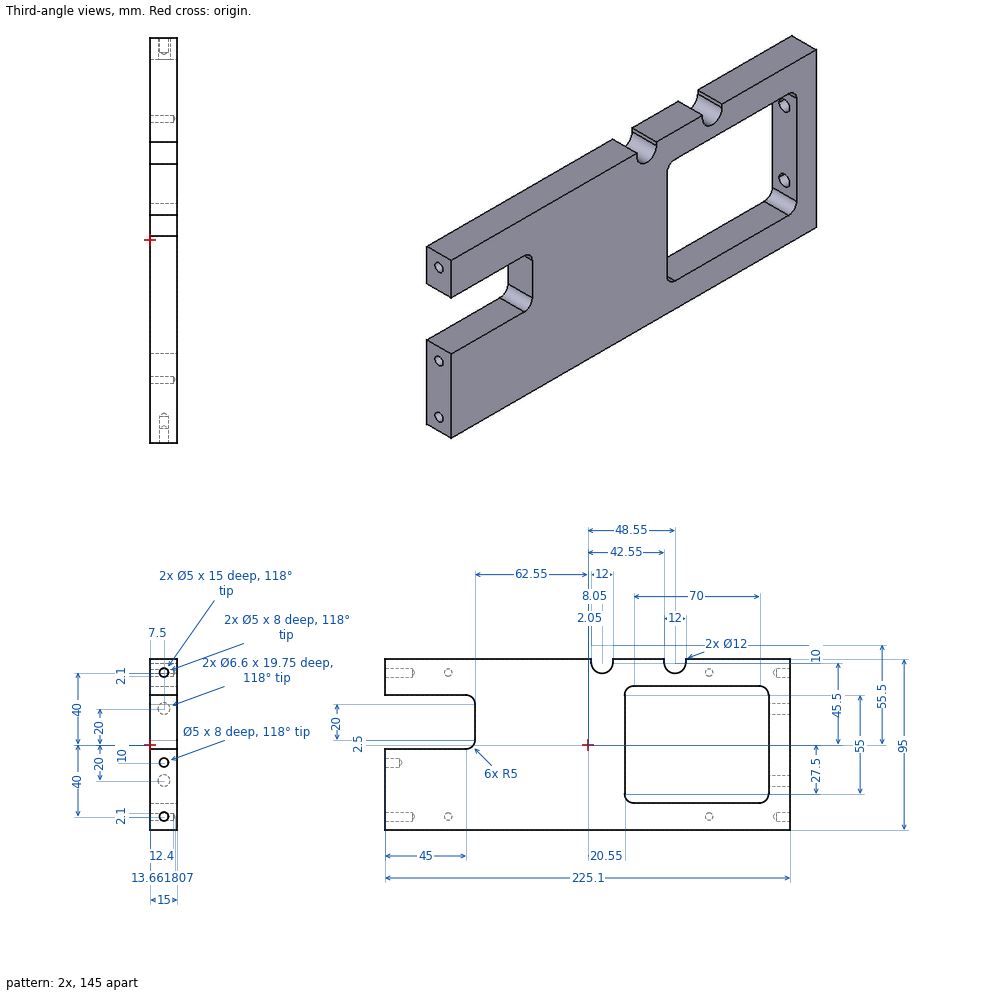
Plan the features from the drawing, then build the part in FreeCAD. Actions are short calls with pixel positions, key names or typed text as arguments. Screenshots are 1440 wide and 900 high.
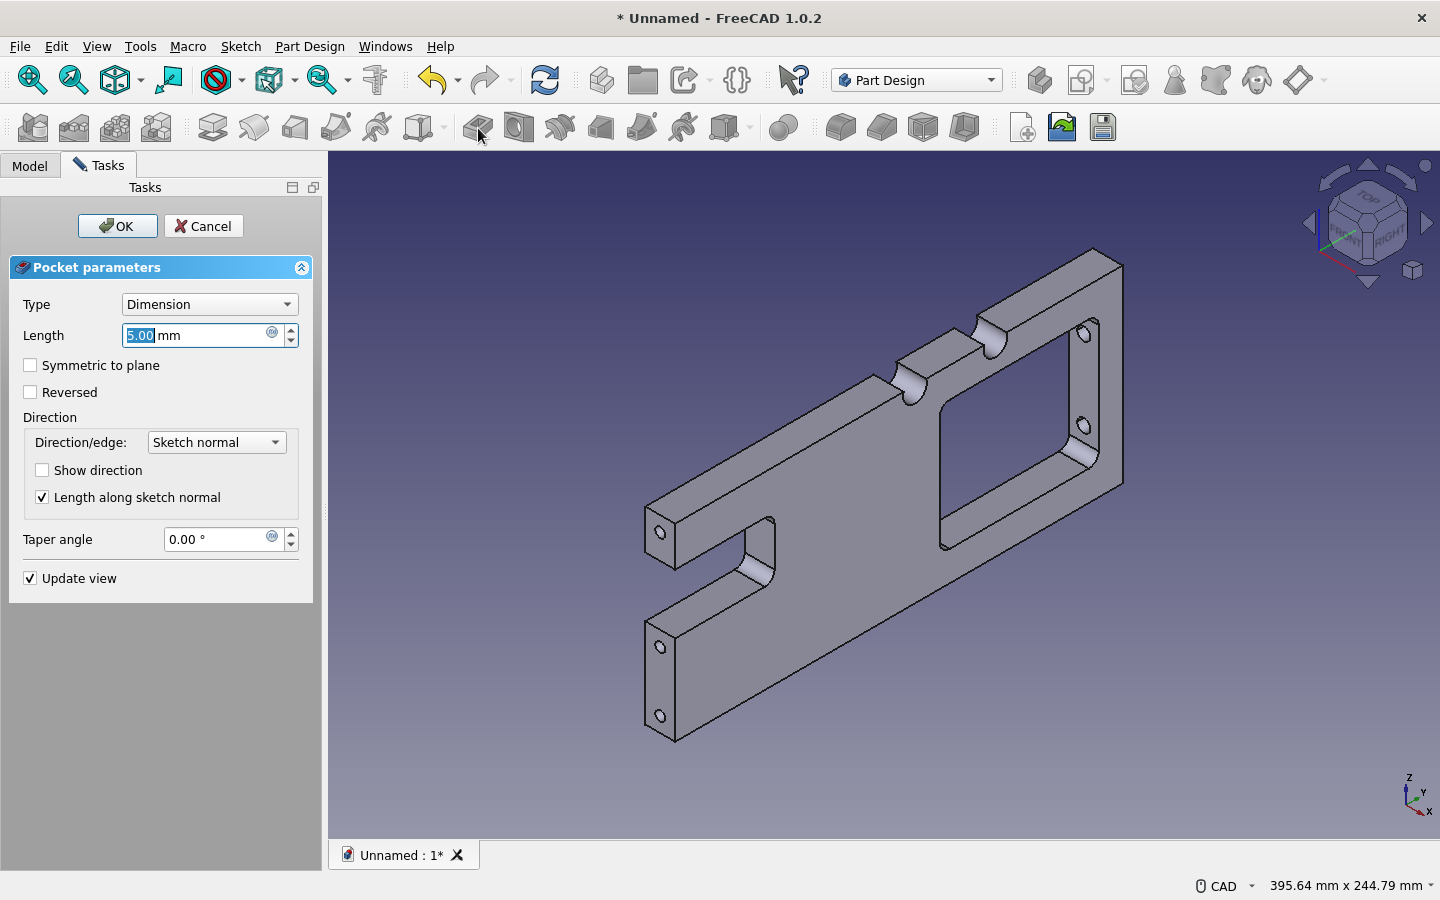
click(210, 304)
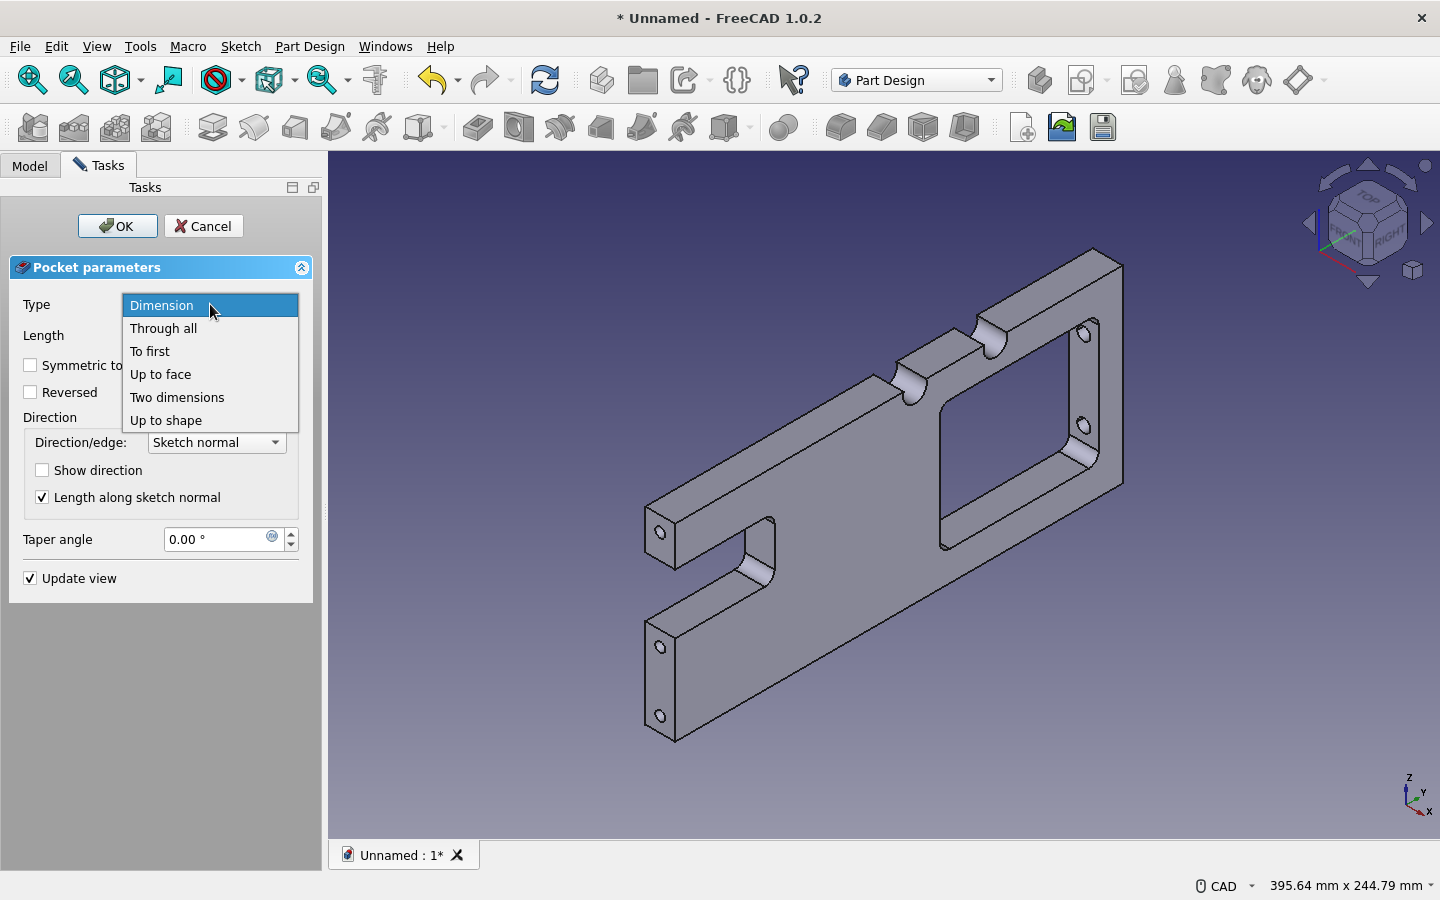
click(208, 328)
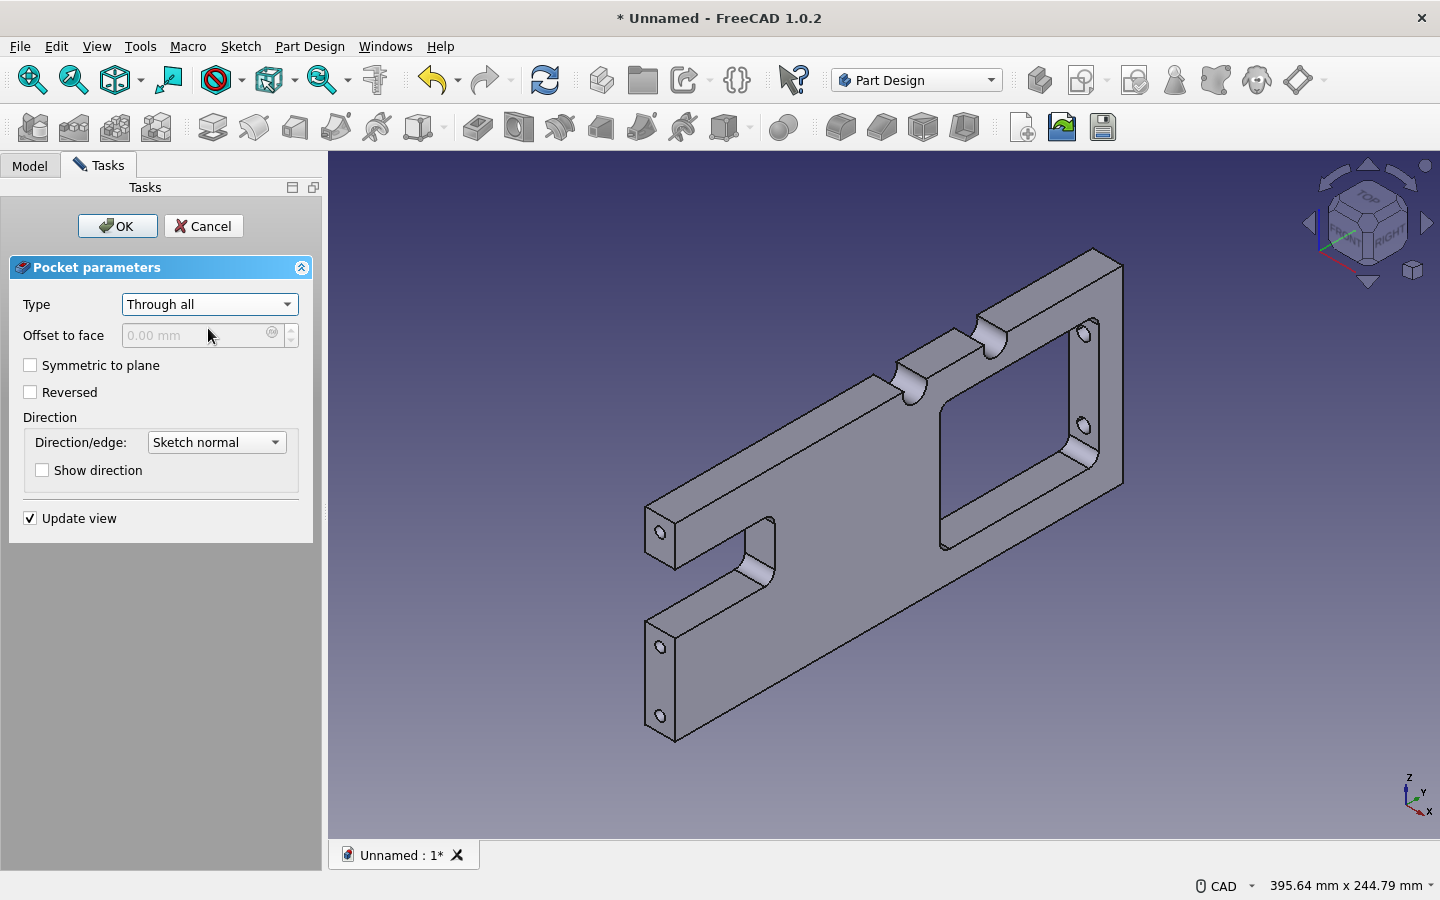
click(31, 392)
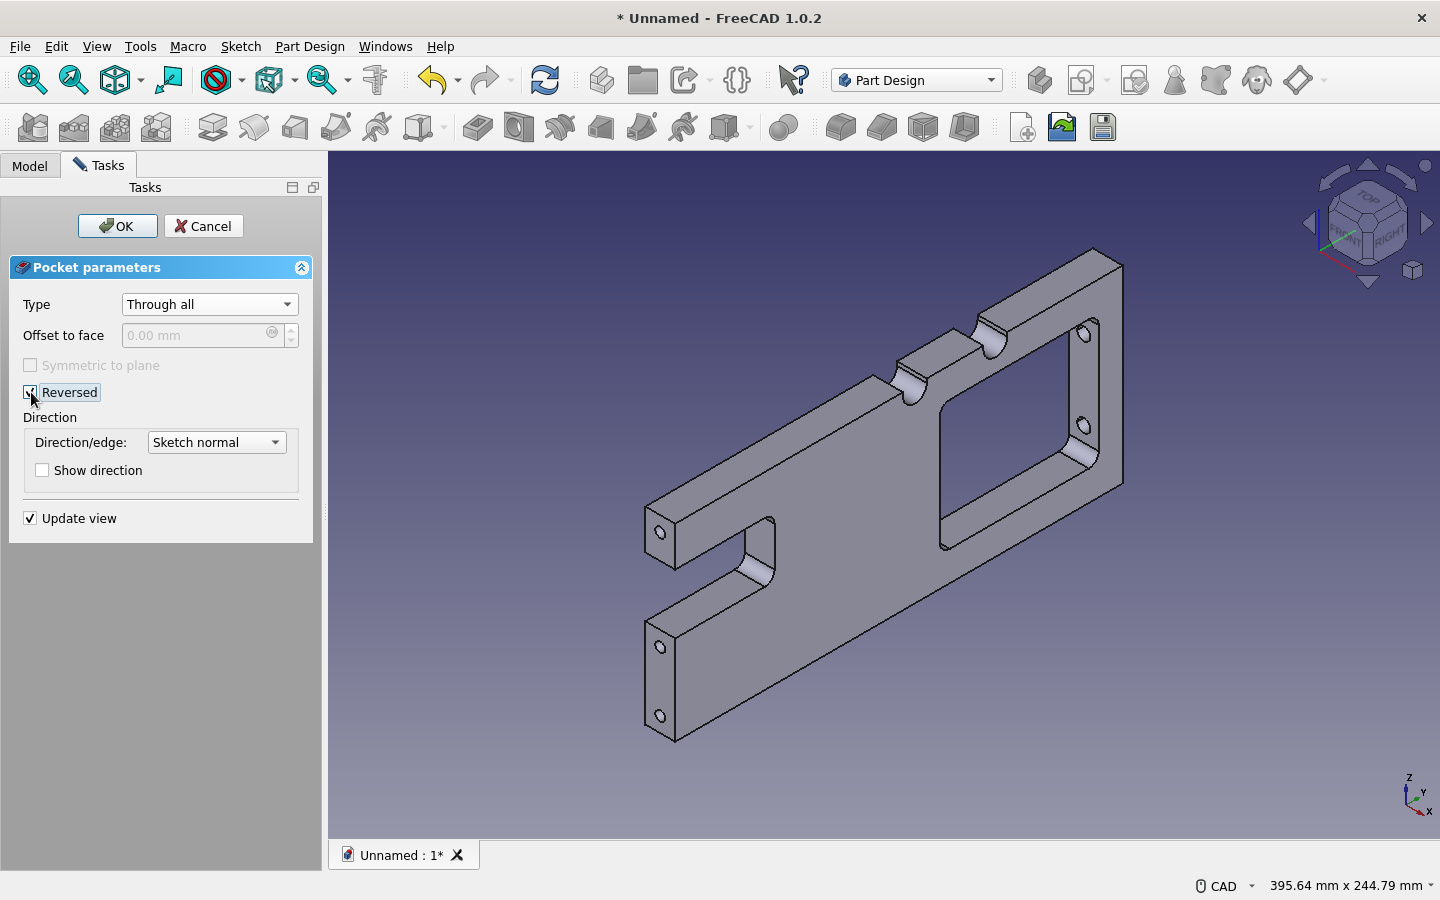
click(118, 226)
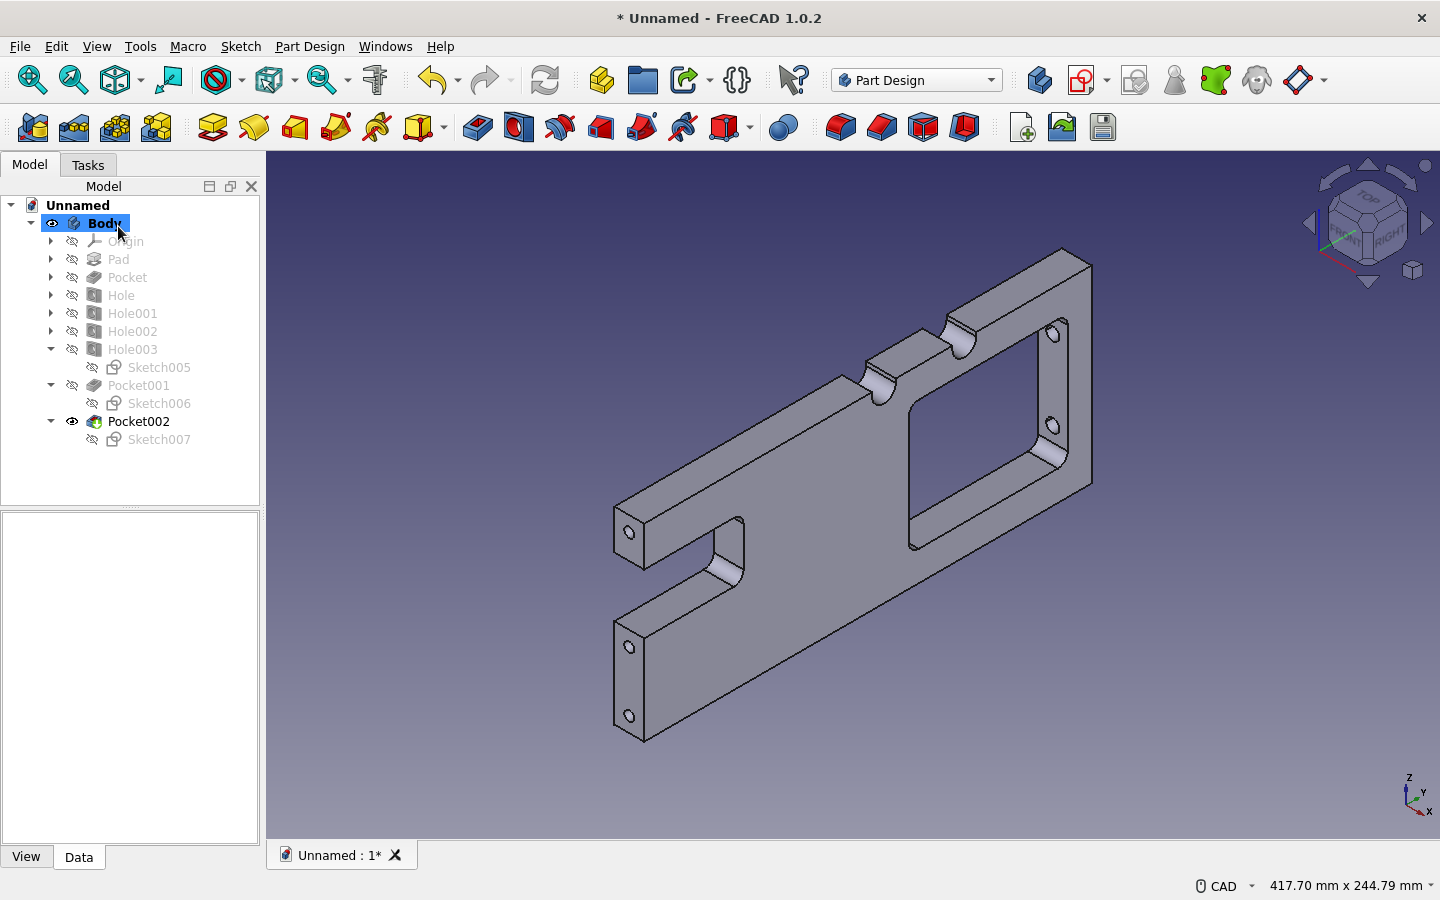
click(51, 241)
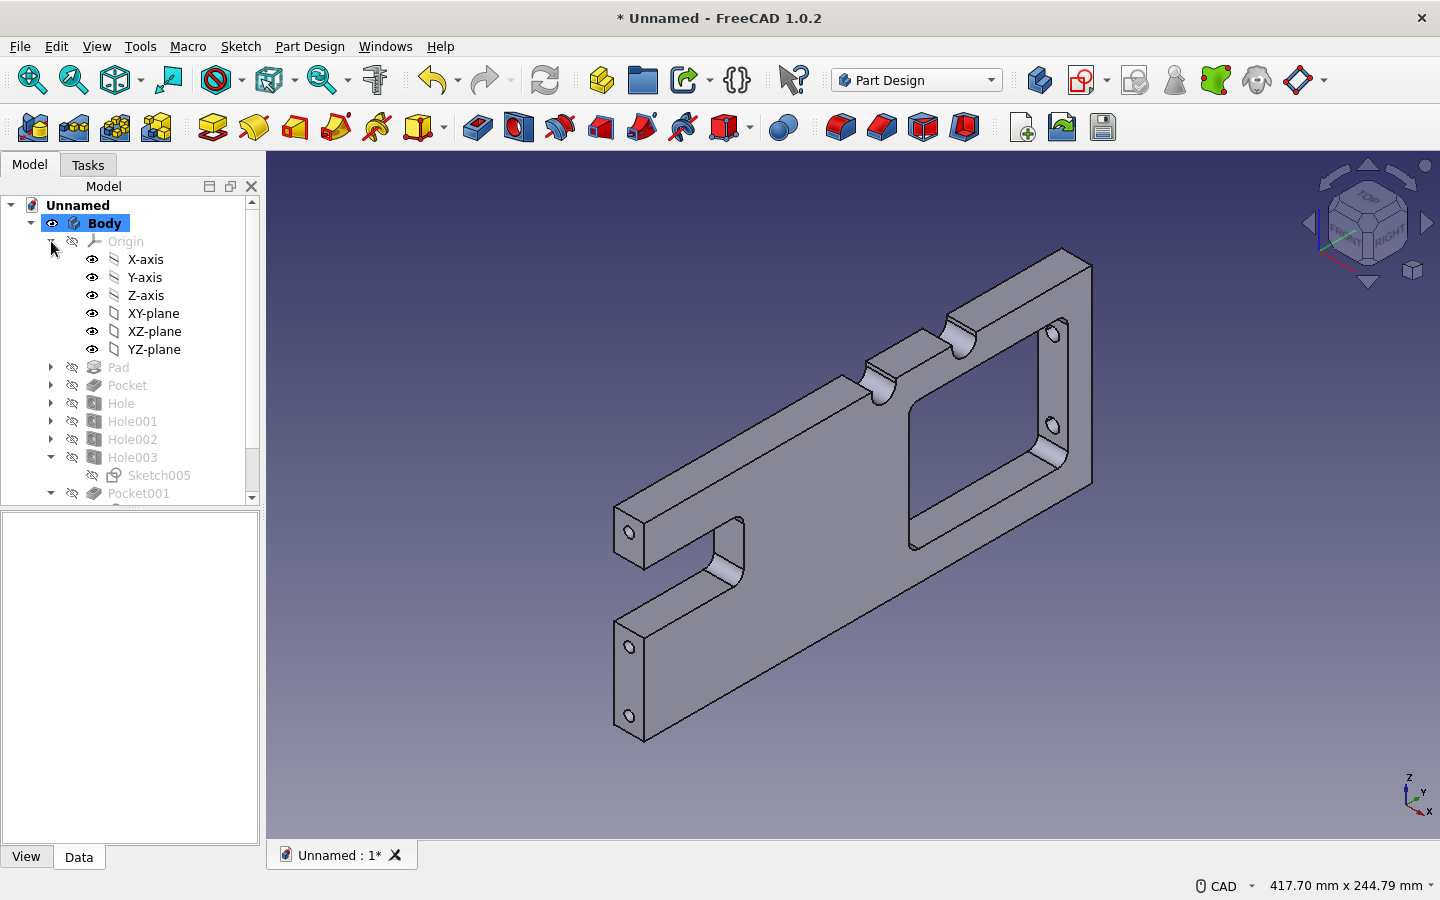
click(137, 331)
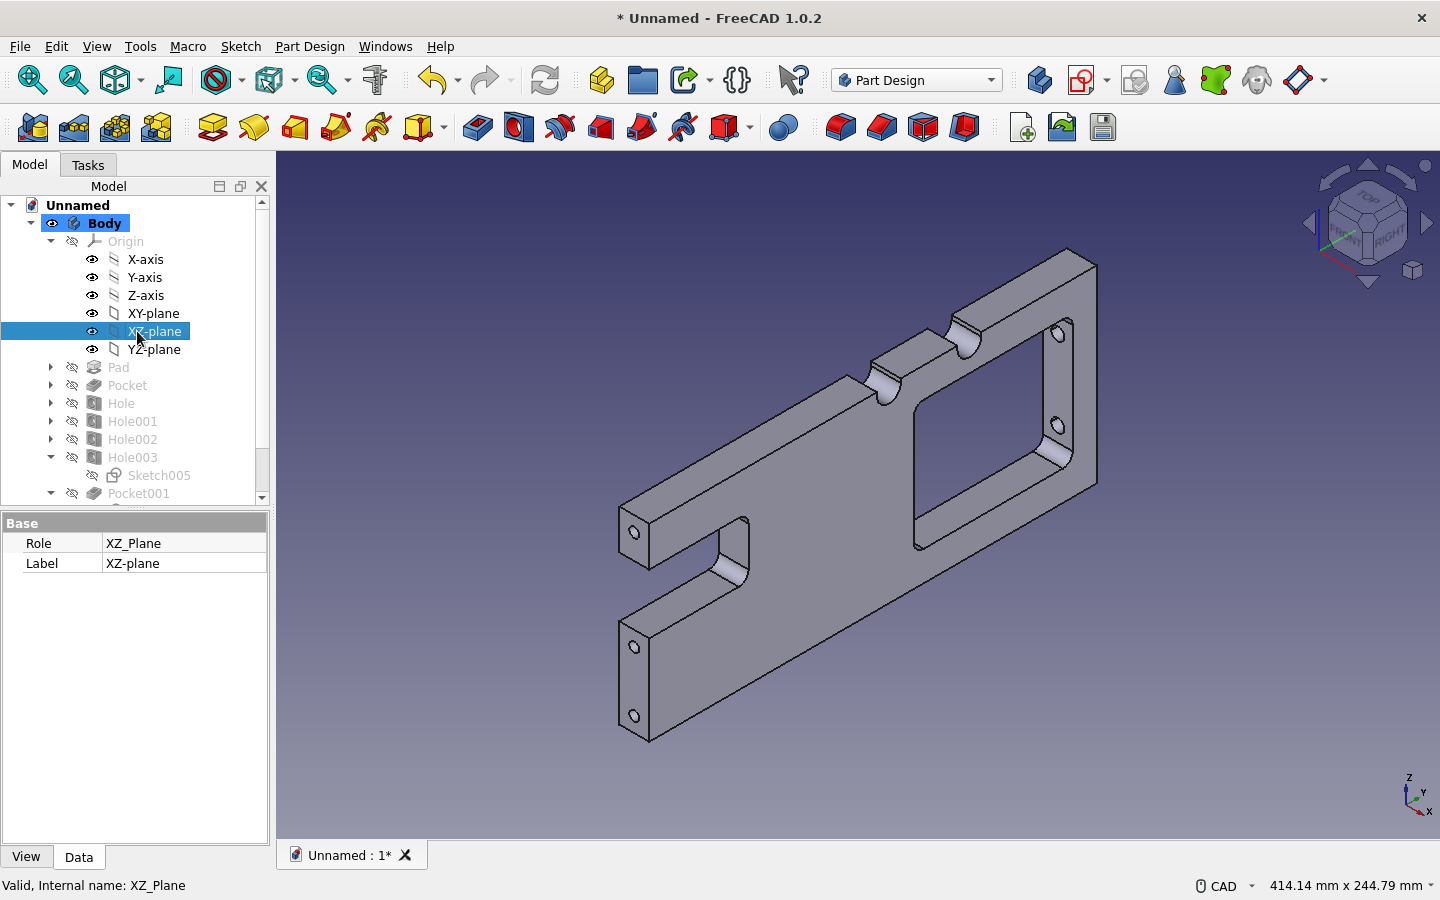
click(1298, 80)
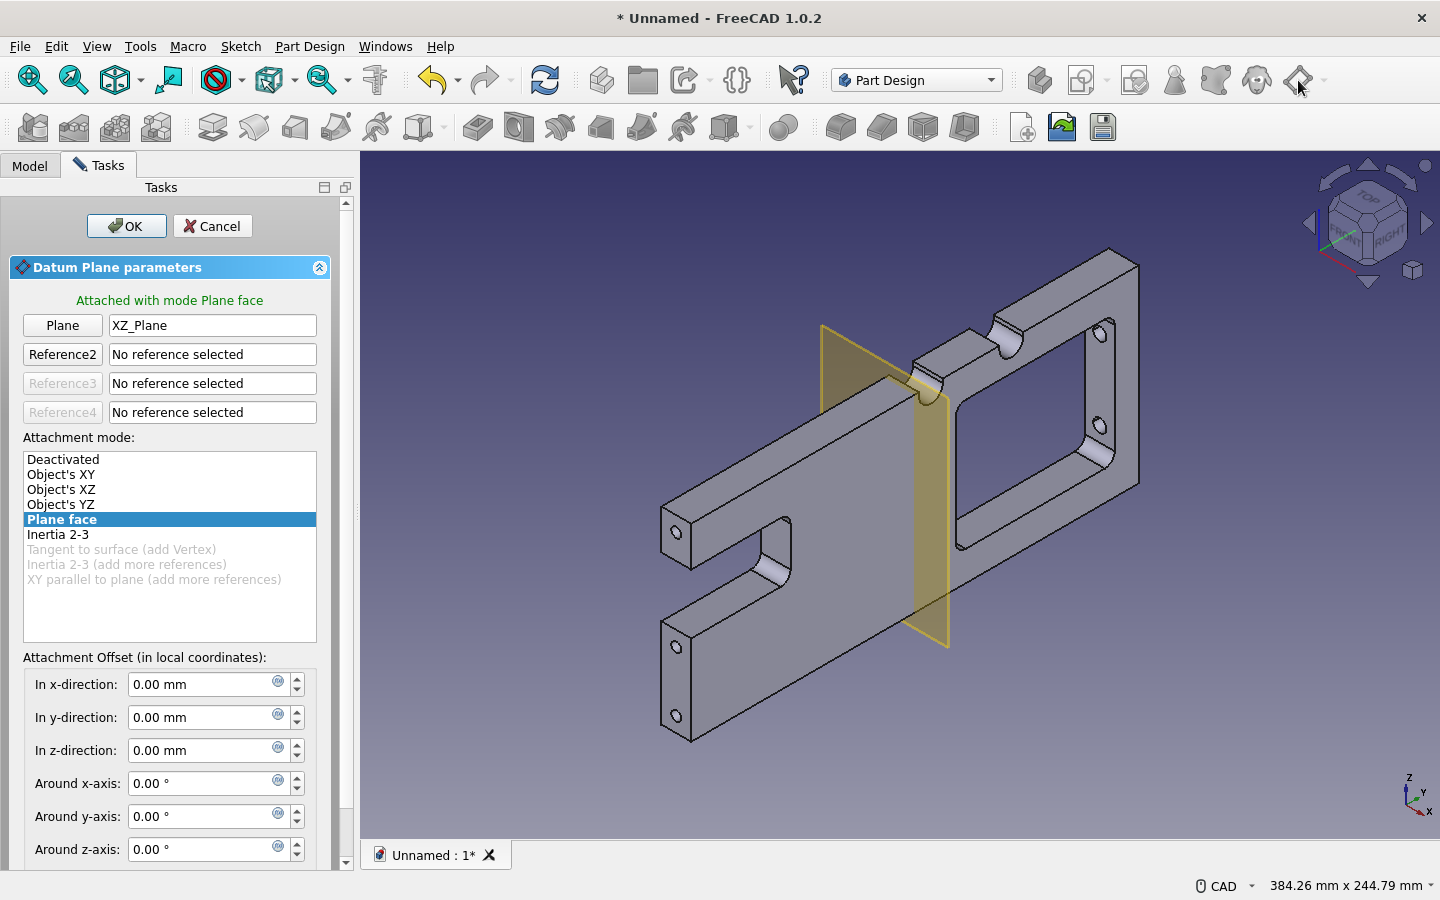
triple_click(210, 750)